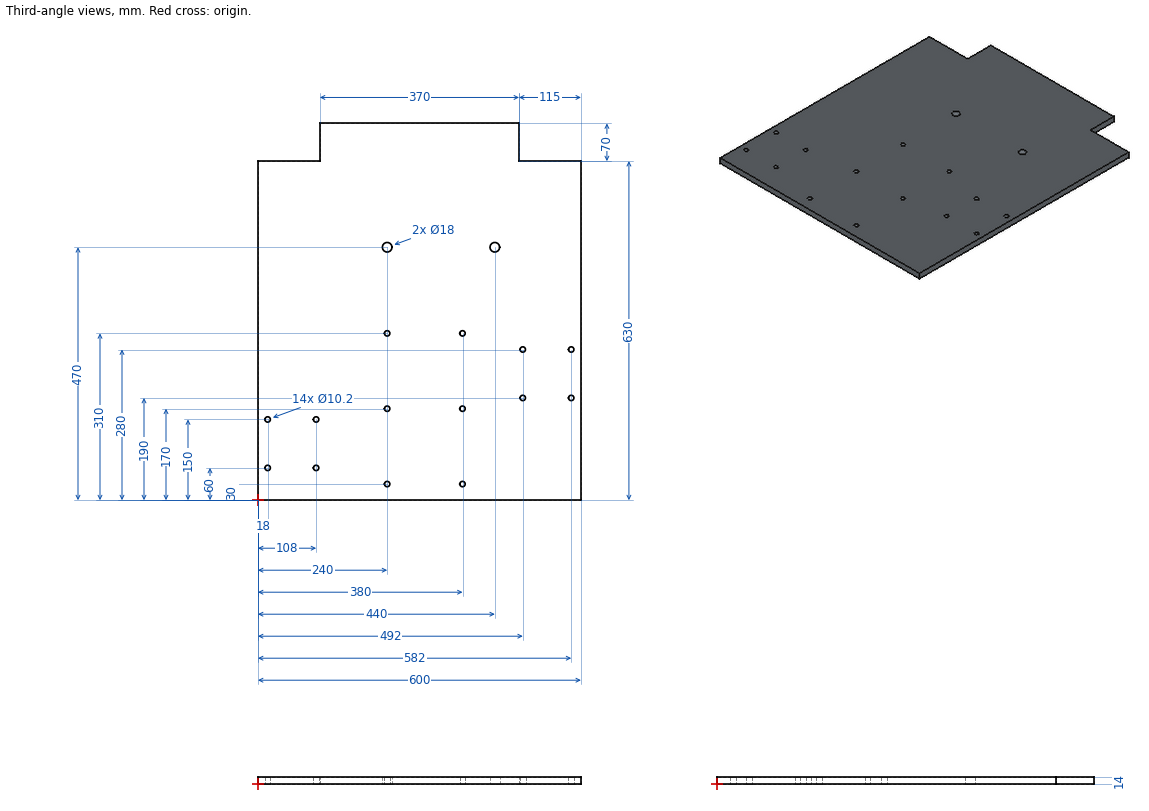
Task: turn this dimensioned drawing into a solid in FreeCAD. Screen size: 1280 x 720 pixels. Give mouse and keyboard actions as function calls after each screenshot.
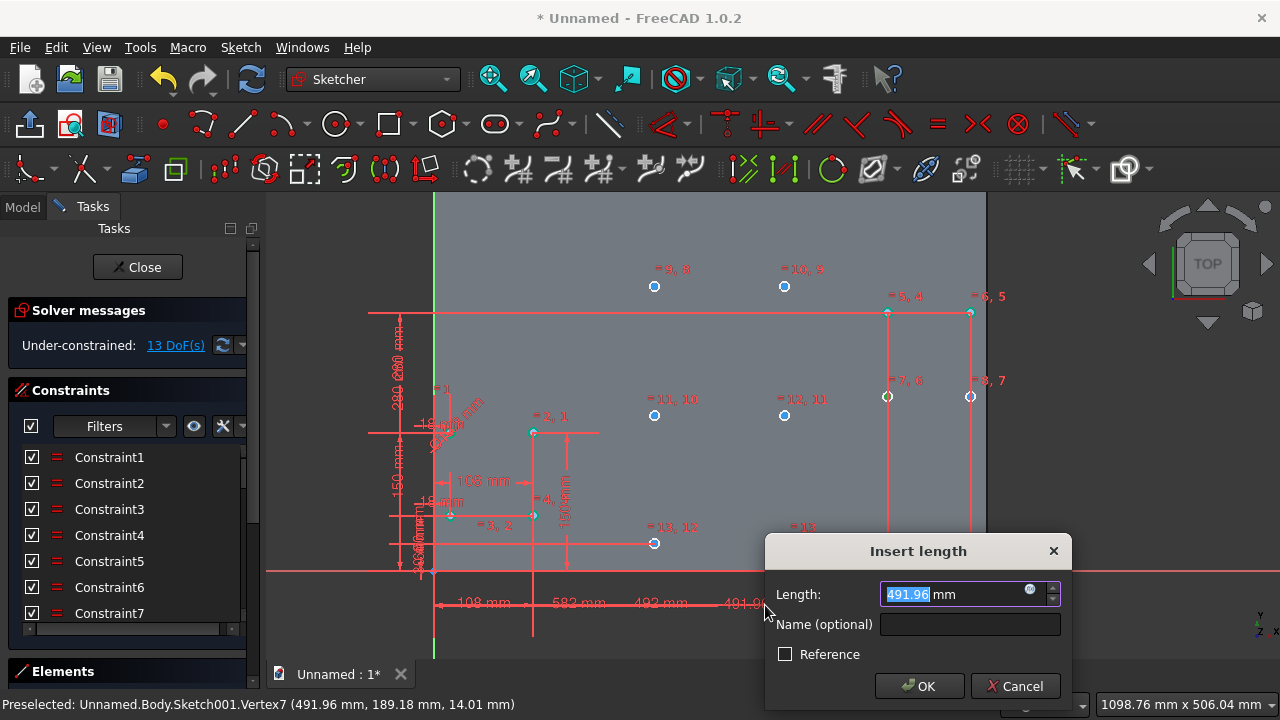
text(492)
key(Return)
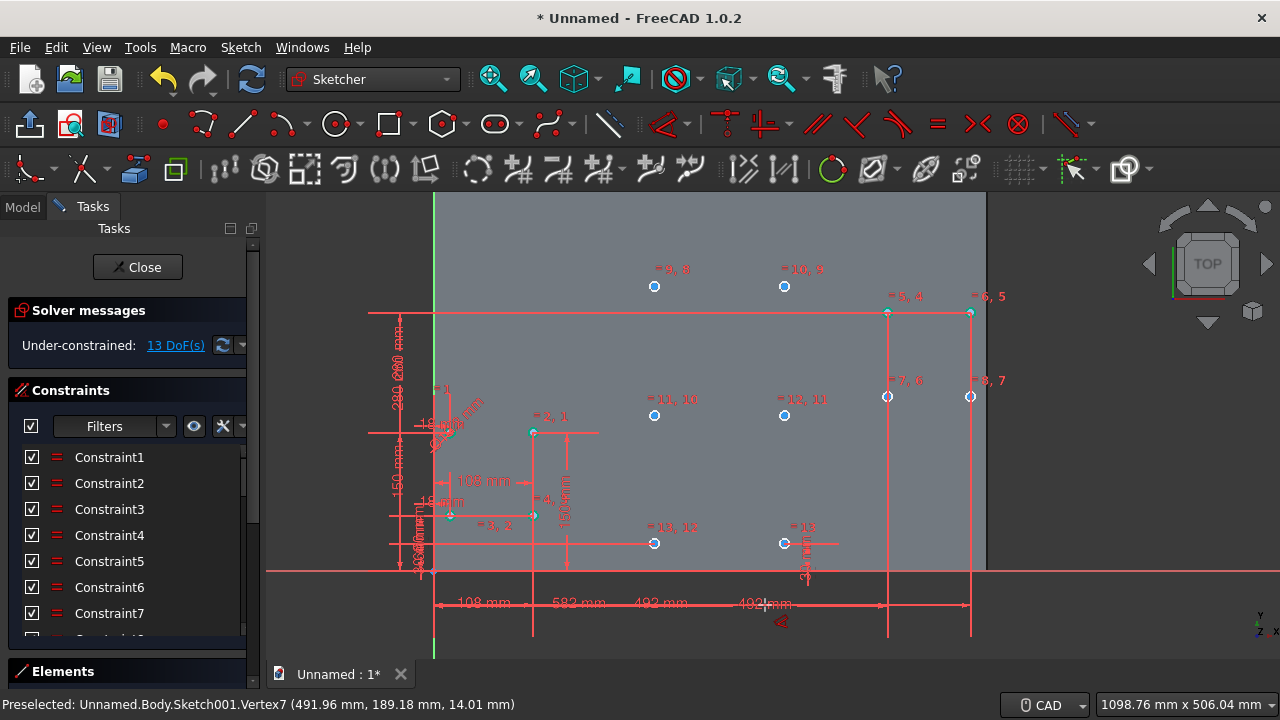
click(888, 397)
click(922, 484)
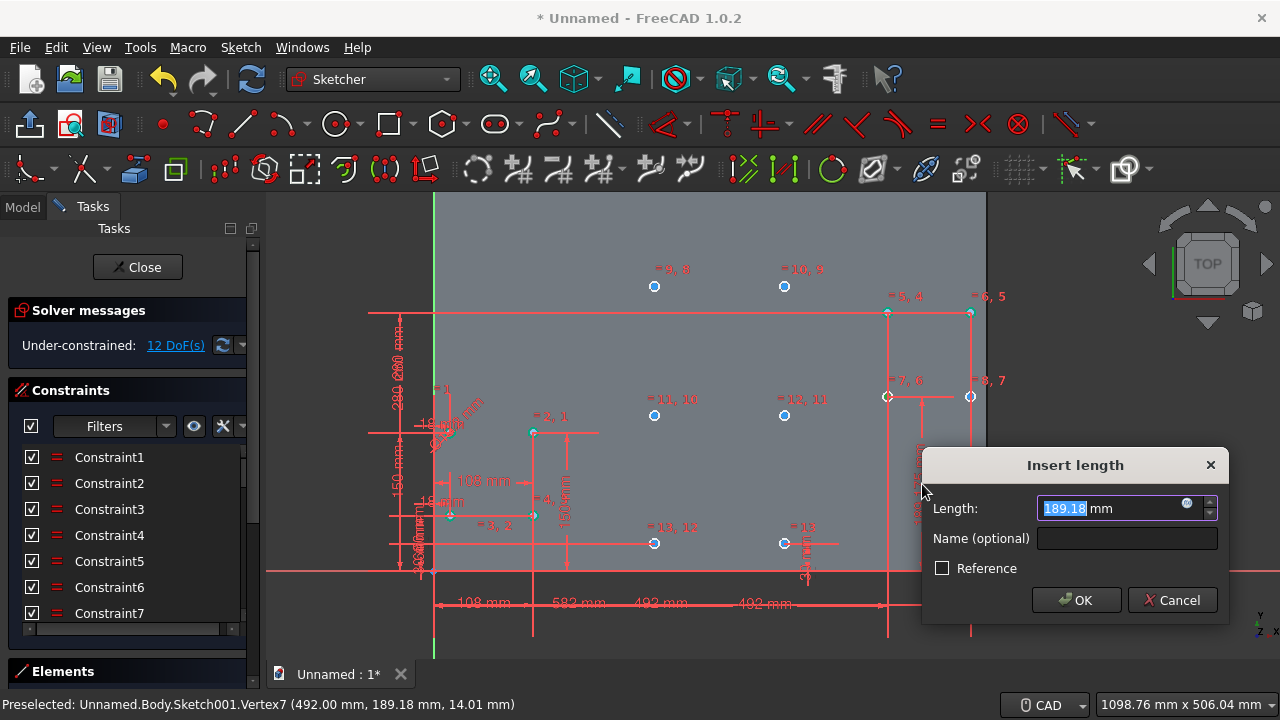
text(190)
key(Return)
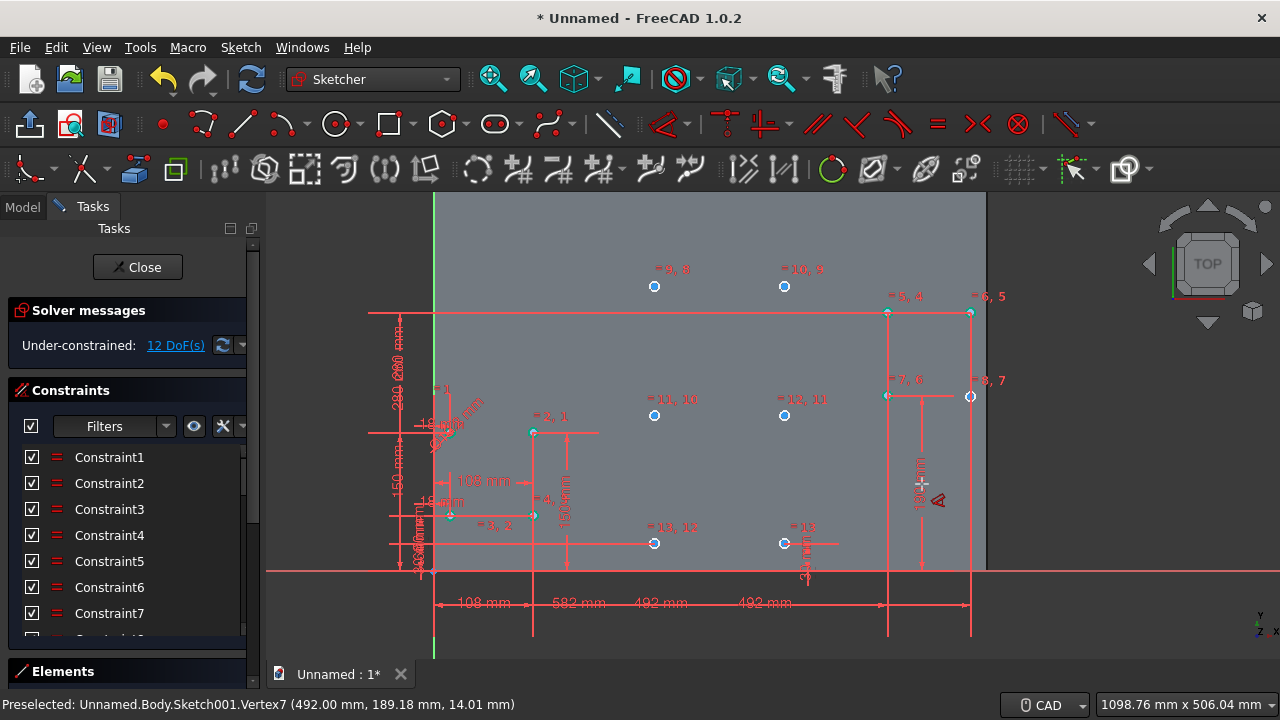
click(971, 397)
click(890, 605)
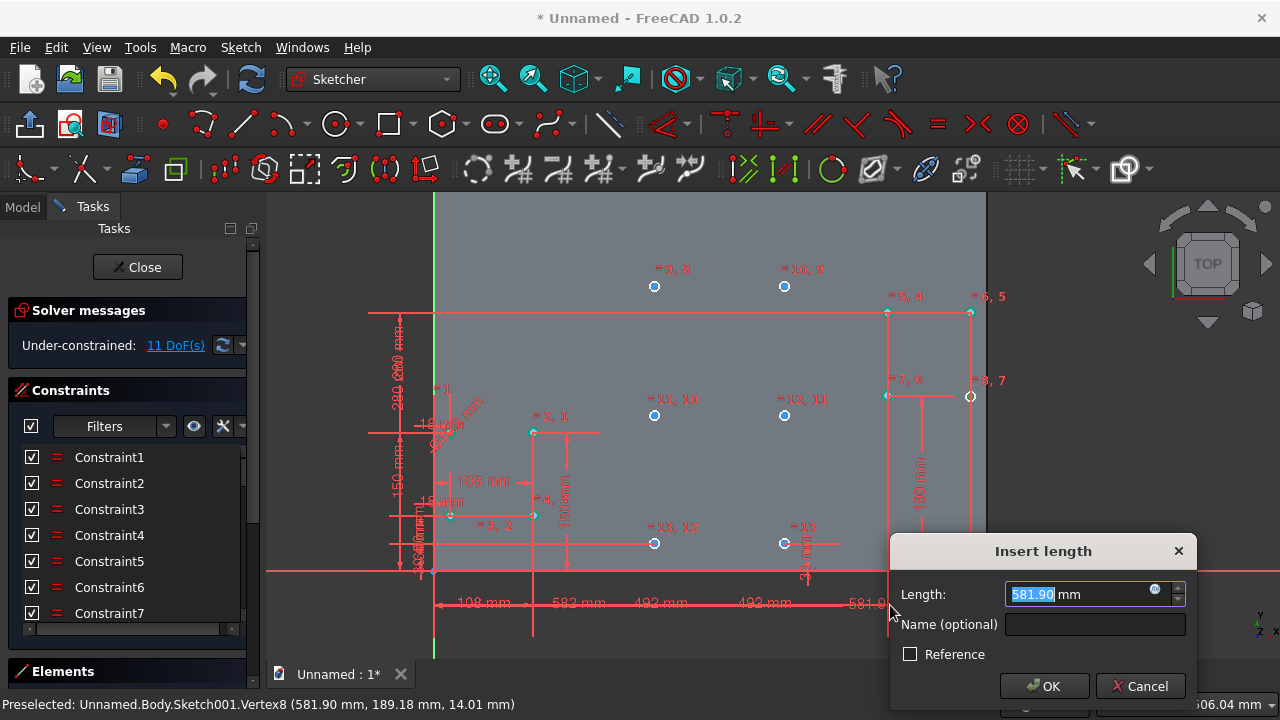
text(582)
key(Return)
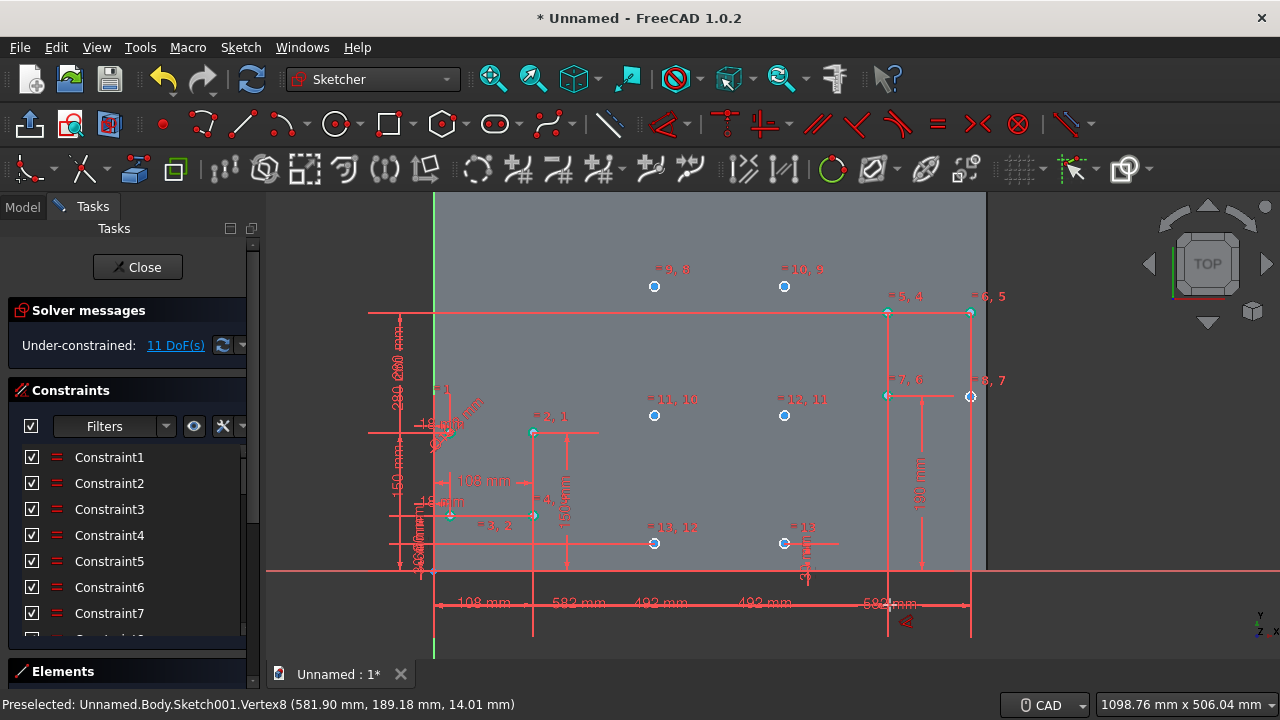
click(971, 397)
click(1005, 484)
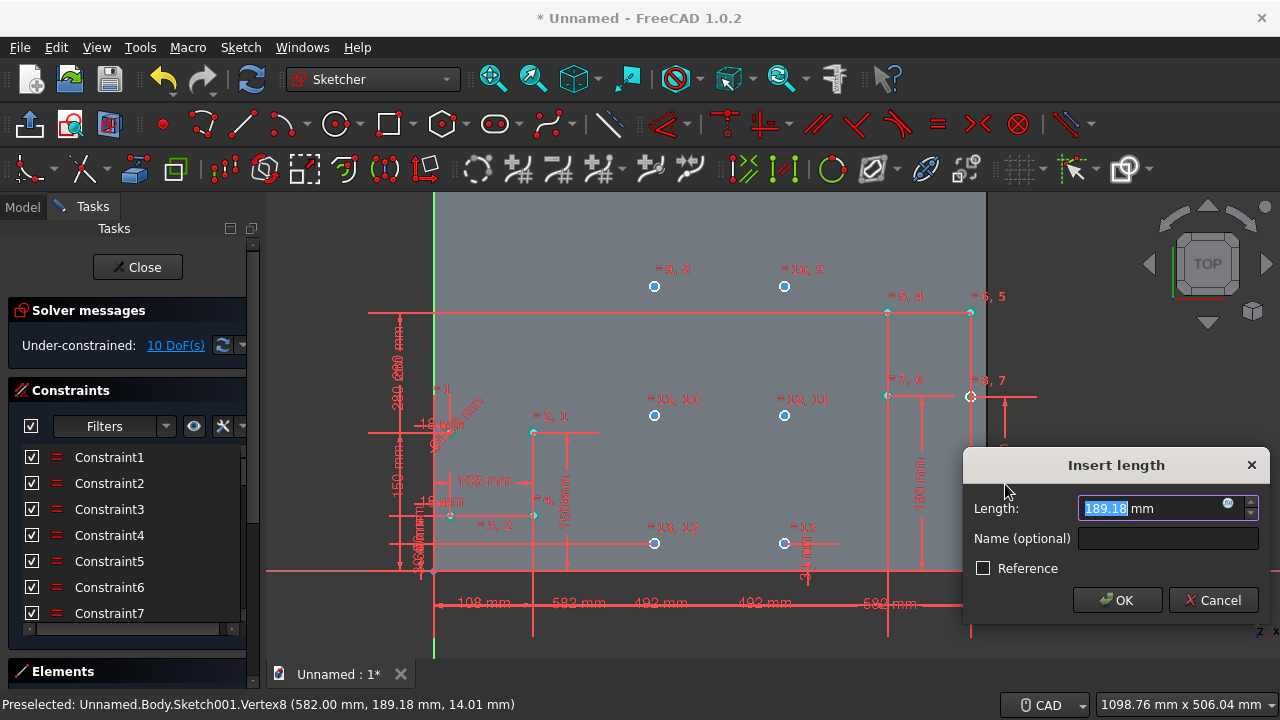
text(190)
key(Return)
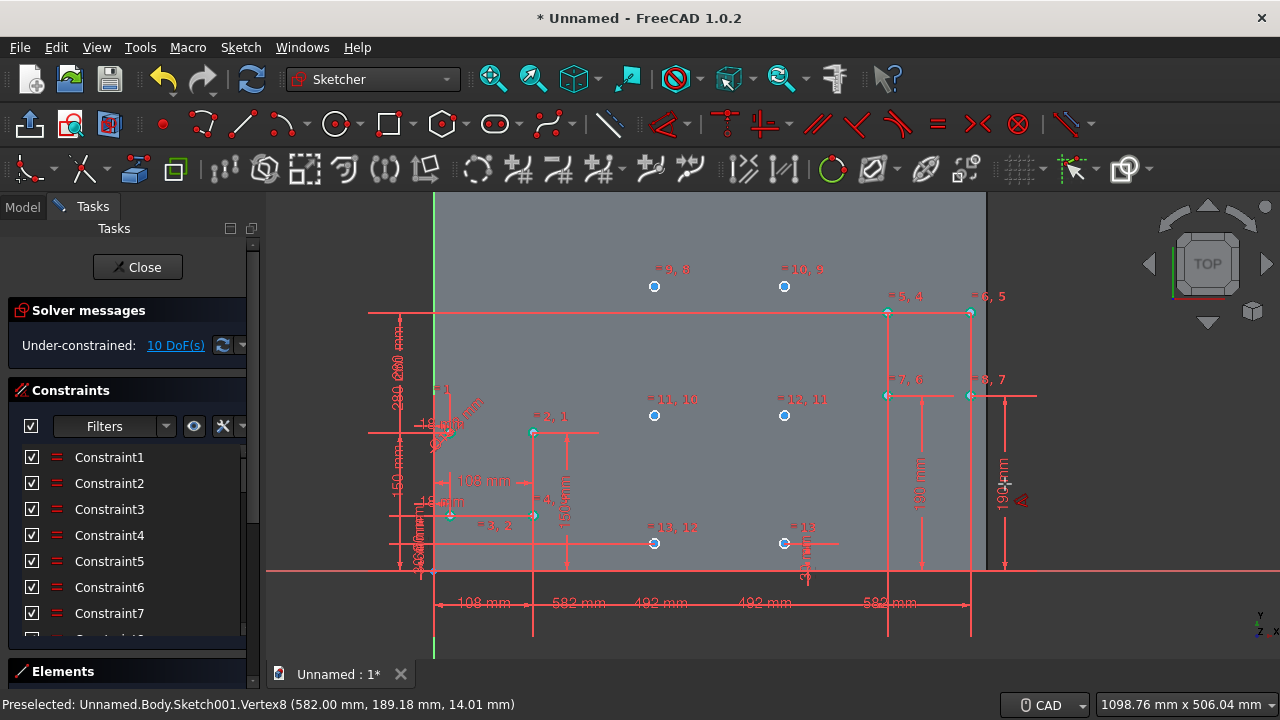
click(655, 286)
click(544, 252)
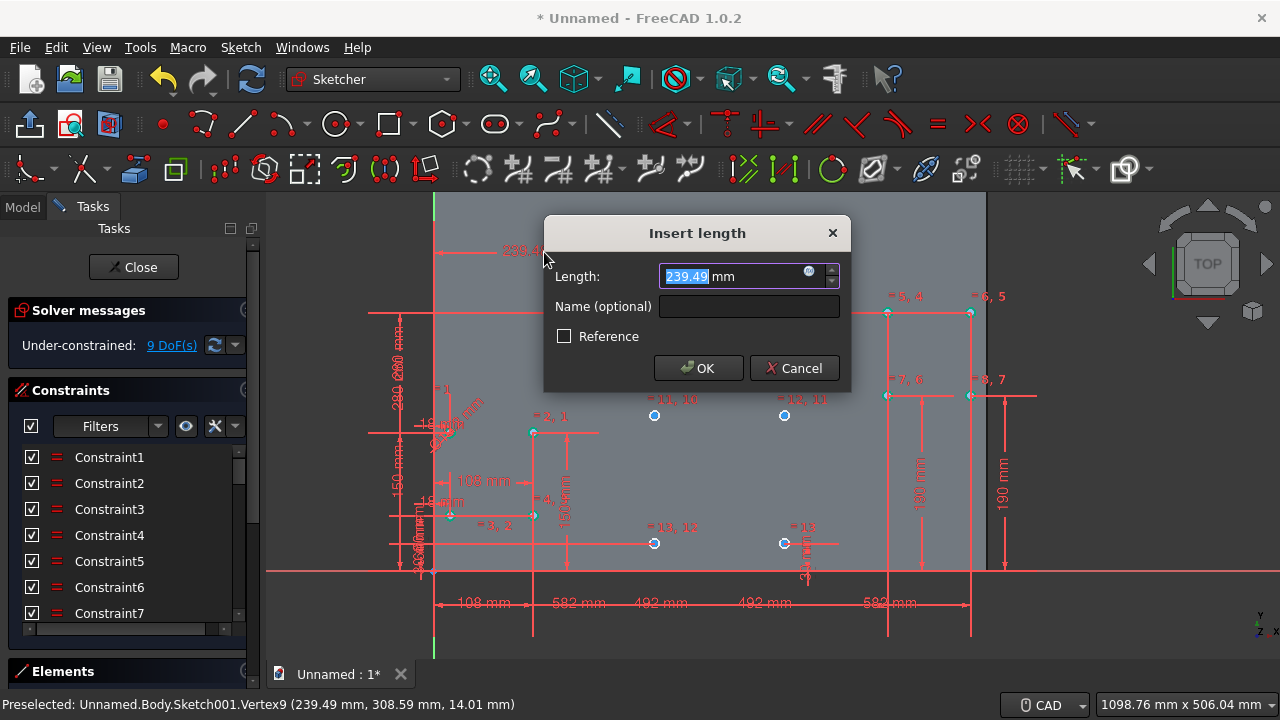
text(240)
key(Return)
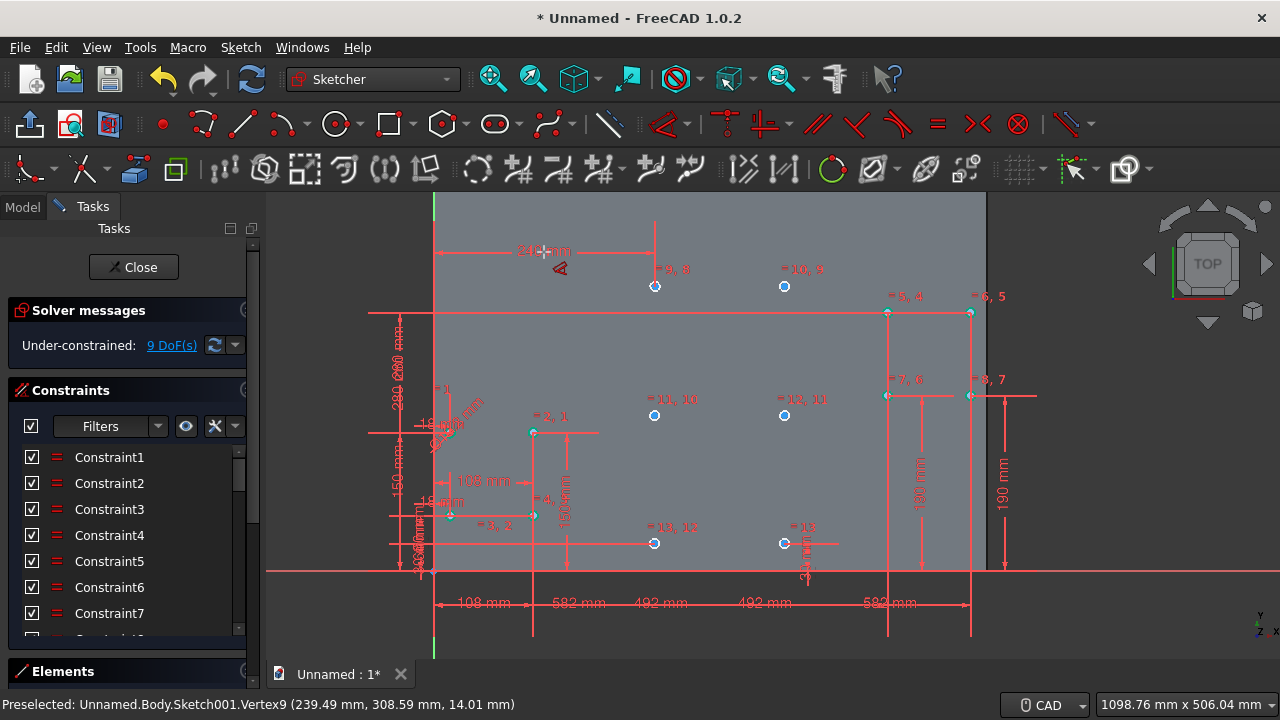
click(655, 286)
click(400, 329)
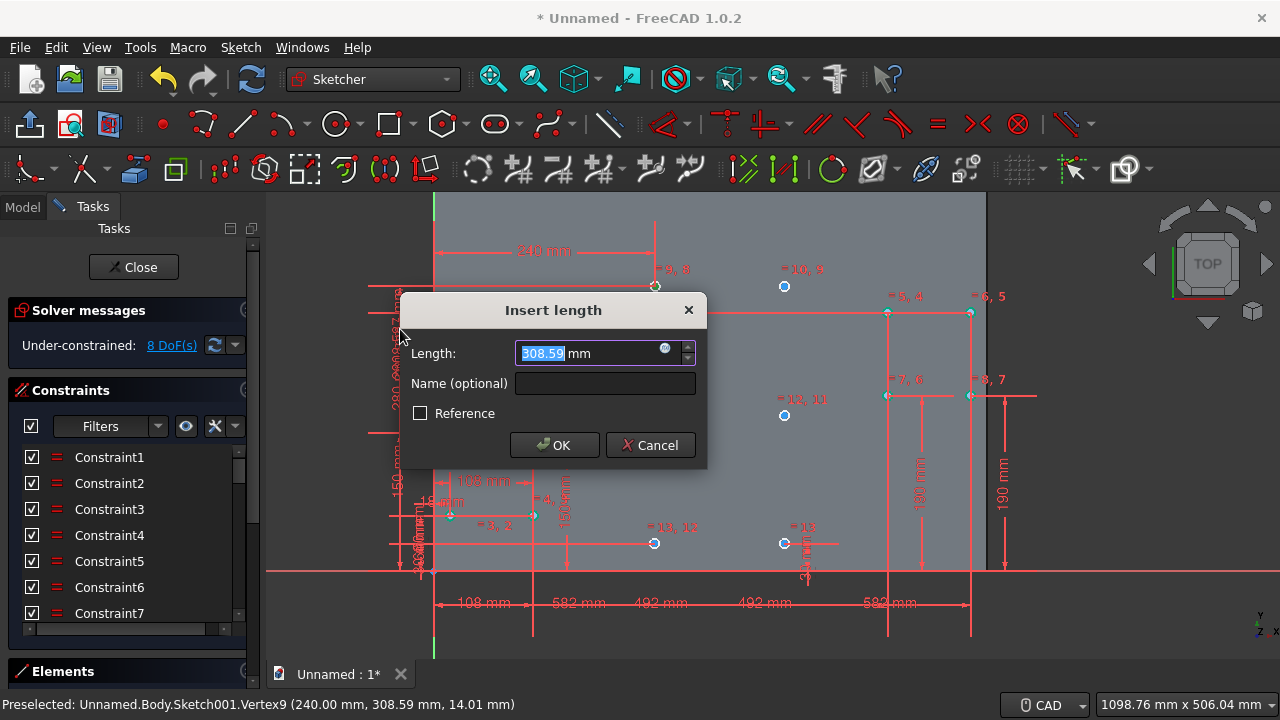
text(310)
key(Return)